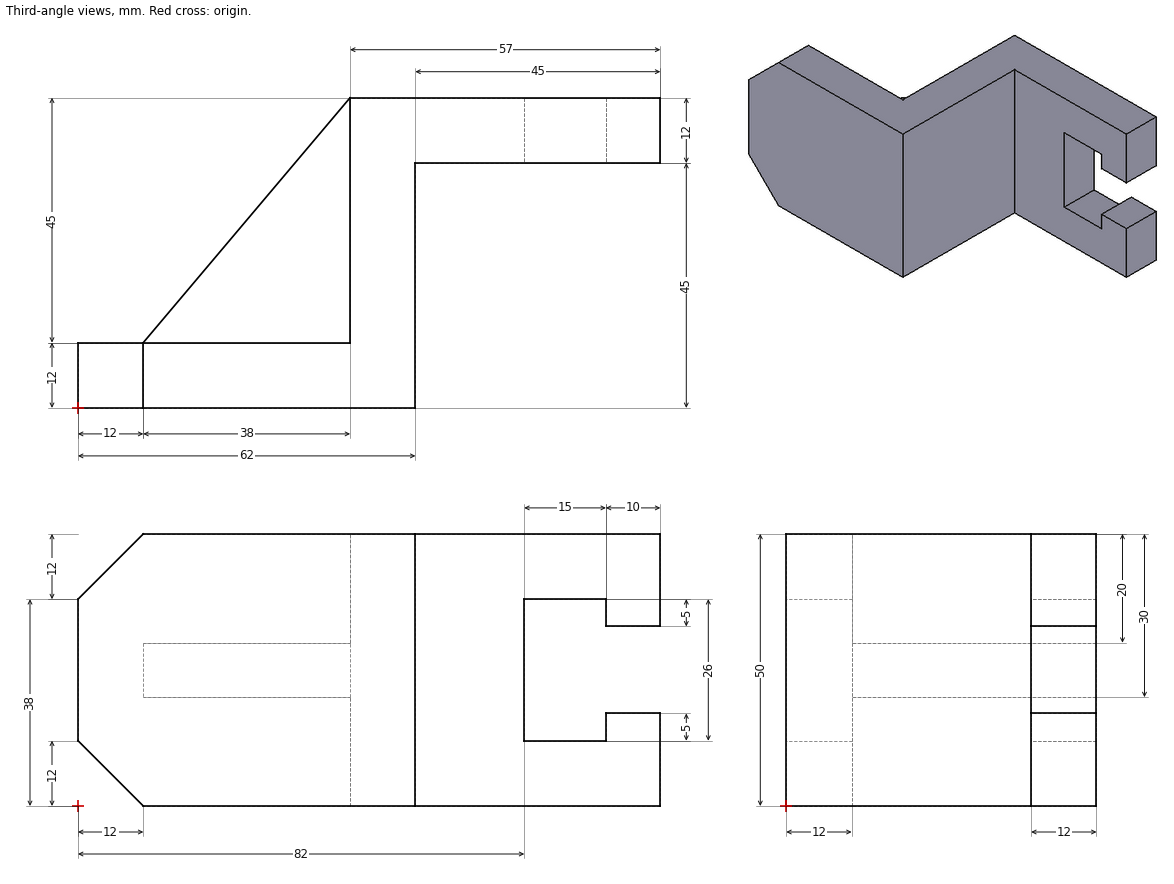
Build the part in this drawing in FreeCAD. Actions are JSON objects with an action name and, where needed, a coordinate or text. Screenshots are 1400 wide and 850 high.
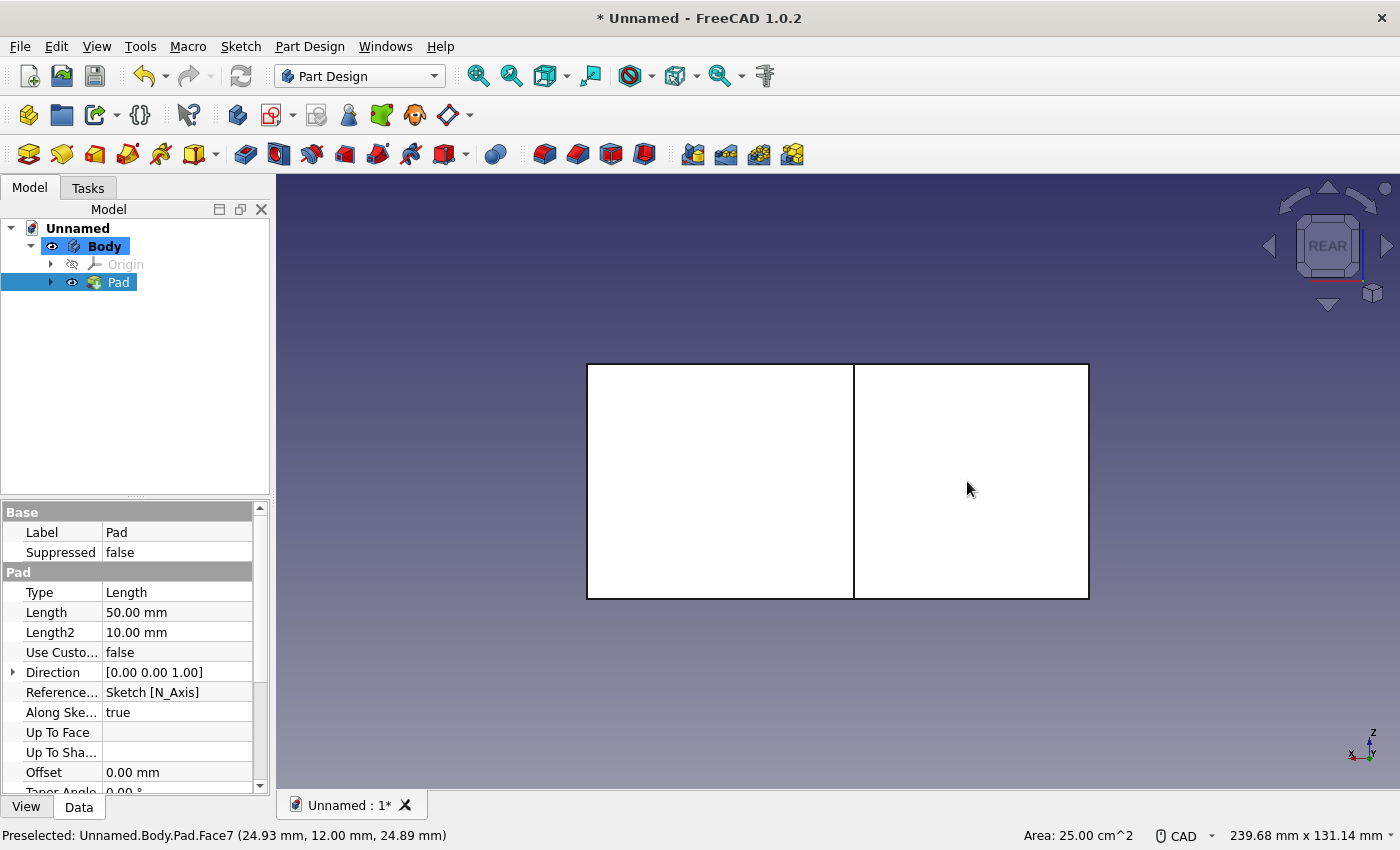
{"action": "left_click", "coordinate": [270, 116]}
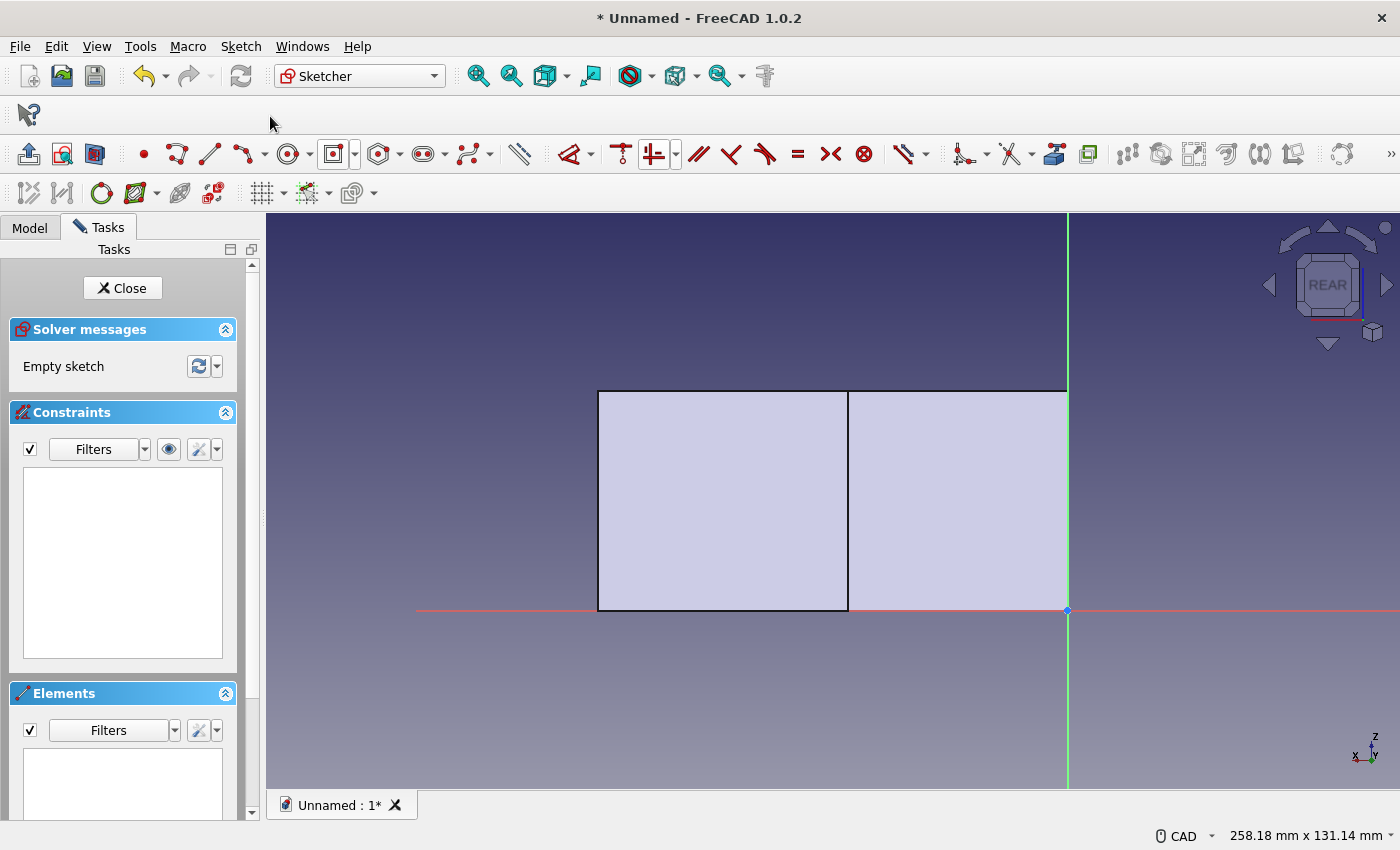
{"action": "scroll", "coordinate": [1235, 501], "scroll_direction": "up", "scroll_amount": 3}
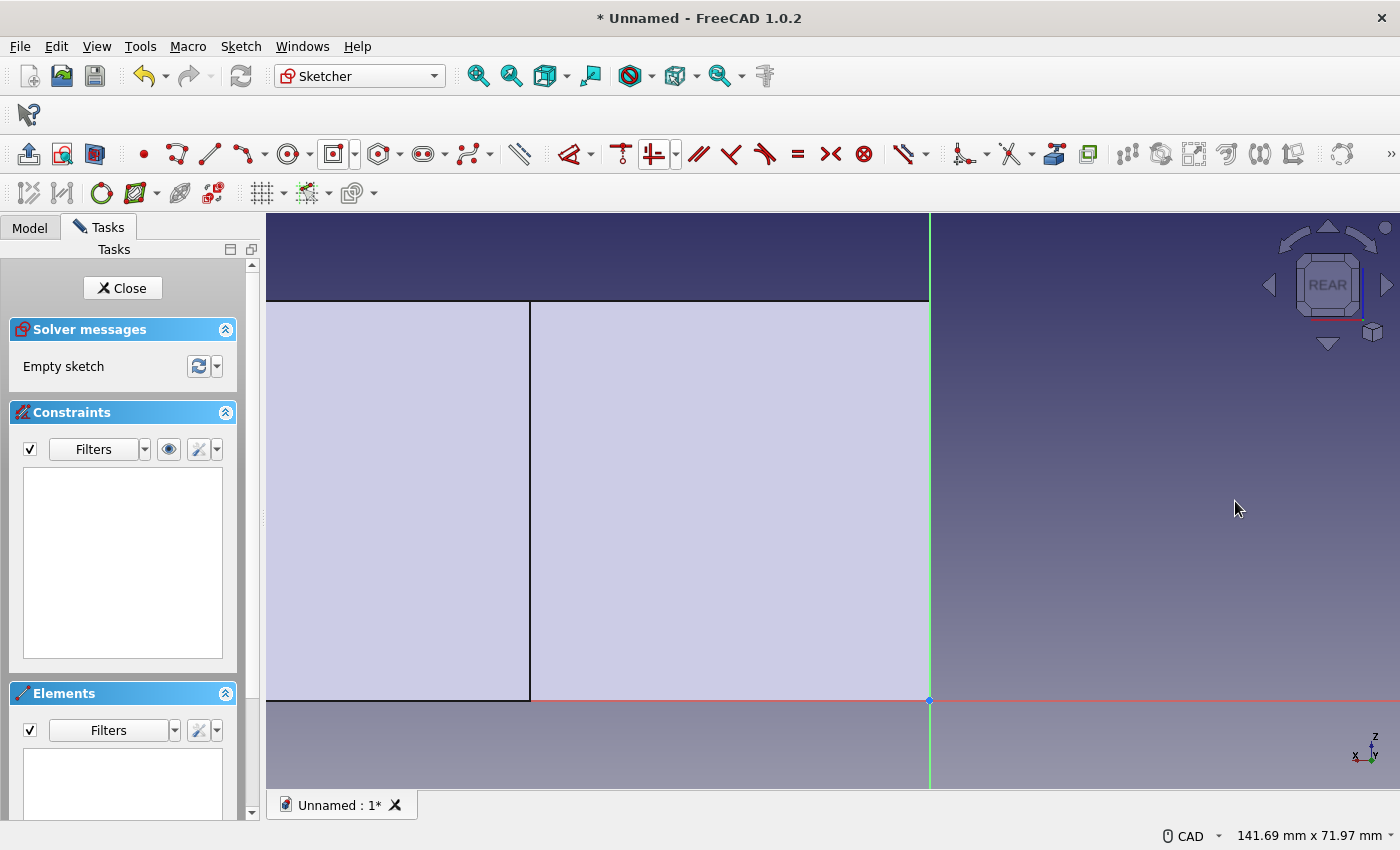
{"action": "left_click", "coordinate": [177, 154]}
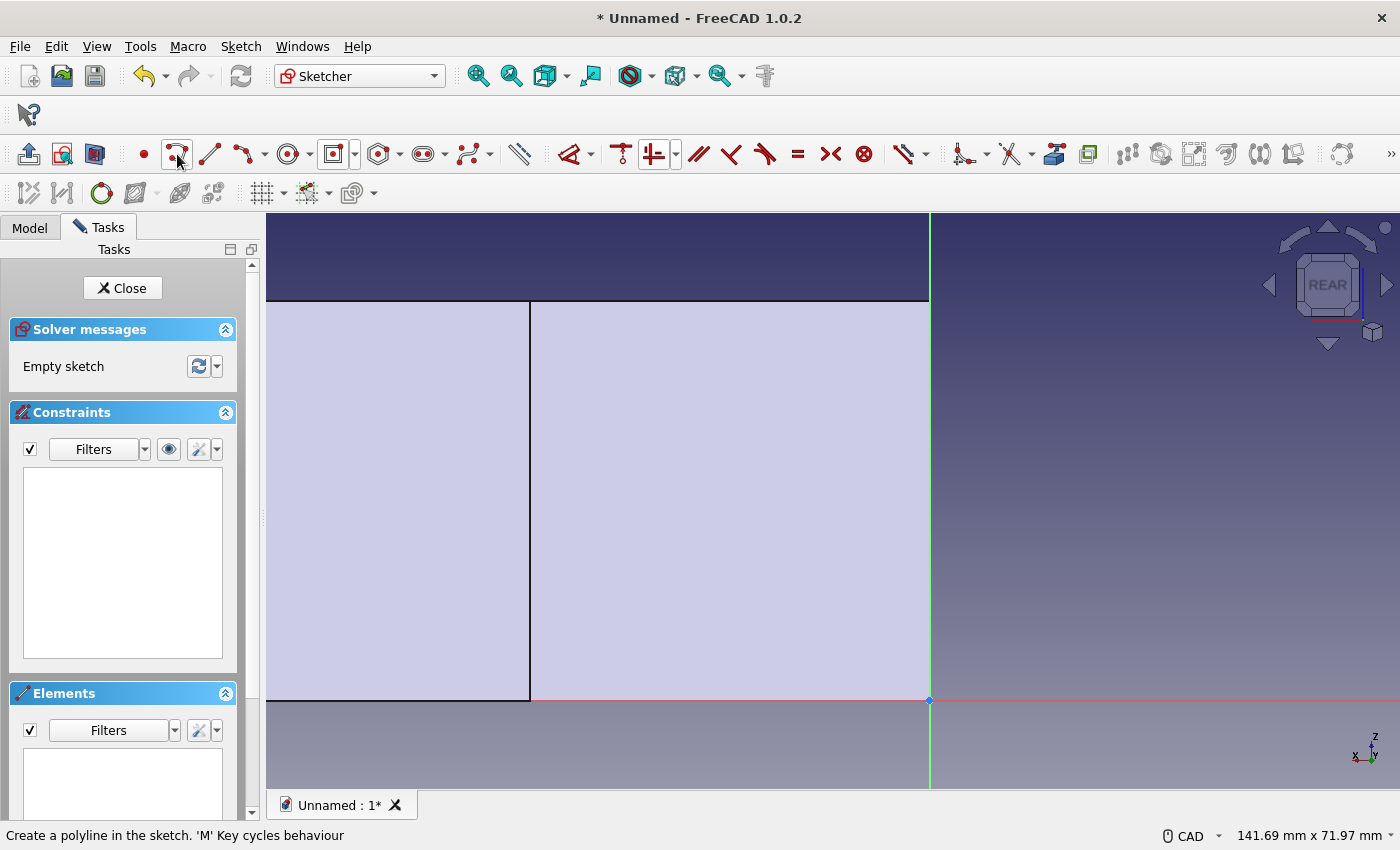
{"action": "left_click", "coordinate": [930, 701]}
{"action": "left_click", "coordinate": [921, 605]}
{"action": "left_click", "coordinate": [834, 692]}
{"action": "left_click", "coordinate": [930, 701]}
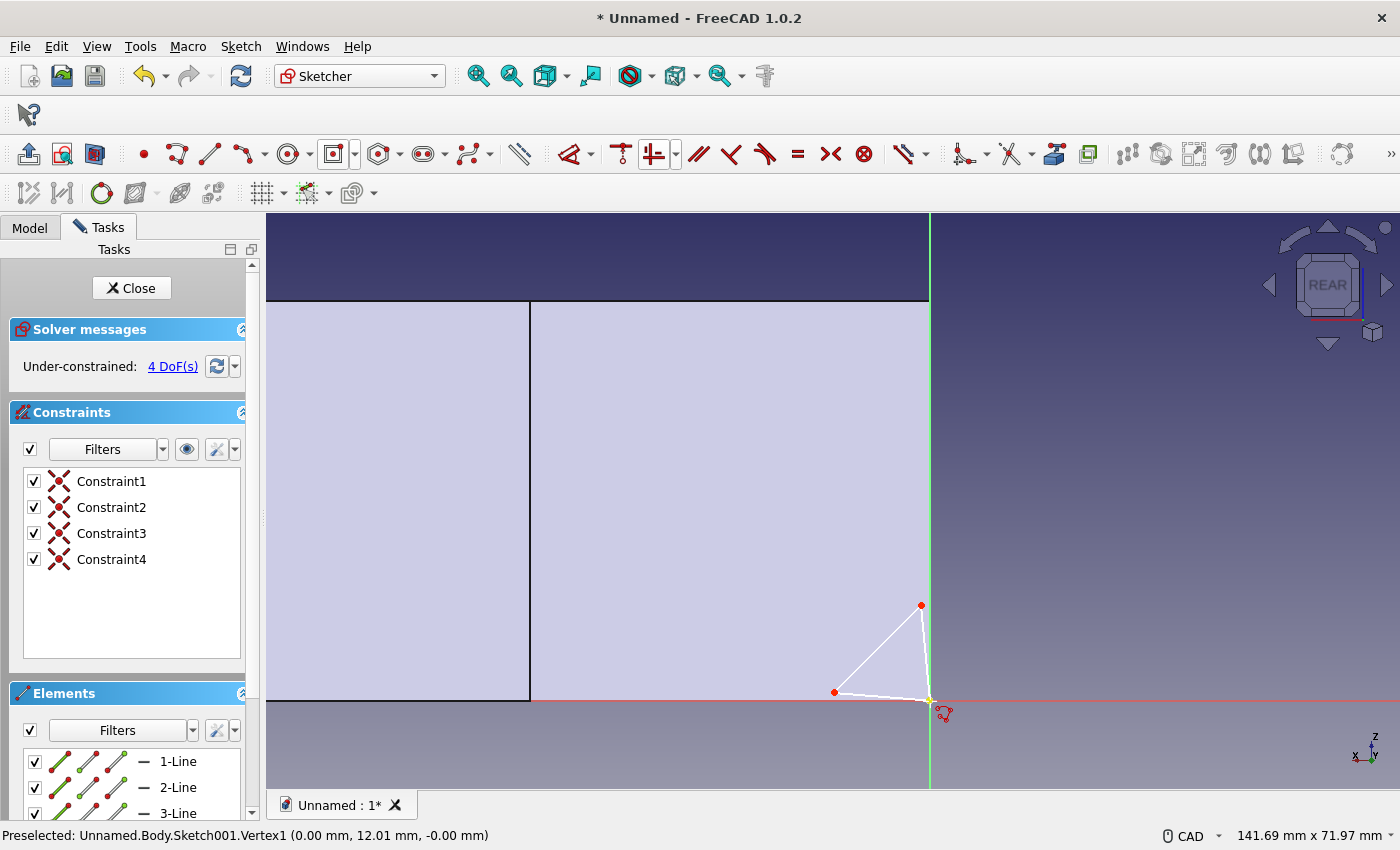
{"action": "left_click", "coordinate": [930, 397]}
{"action": "left_click", "coordinate": [921, 301]}
{"action": "left_click", "coordinate": [834, 301]}
{"action": "left_click", "coordinate": [930, 398]}
{"action": "key", "text": "Escape"}
{"action": "key", "text": "Escape"}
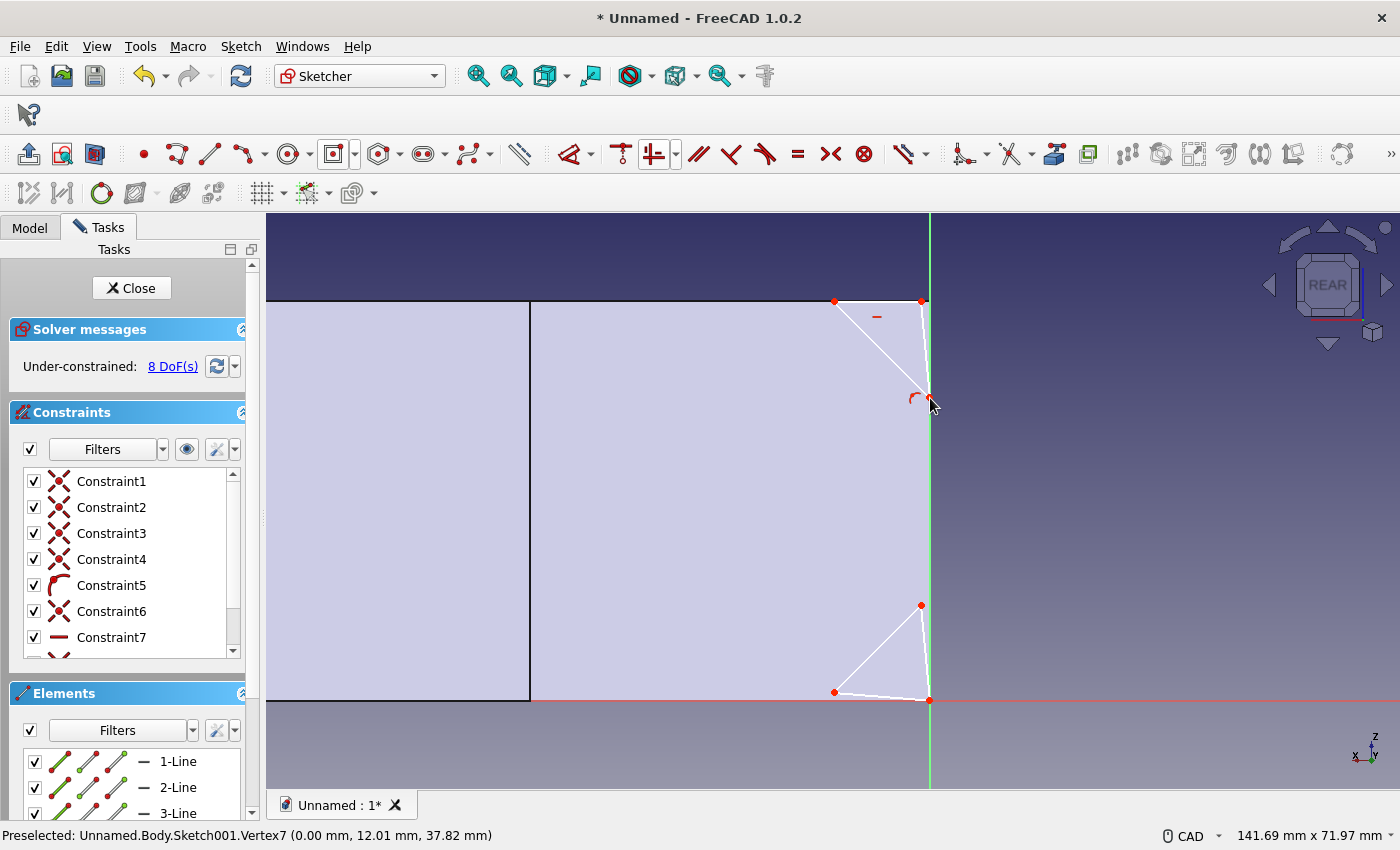
{"action": "left_click", "coordinate": [927, 672]}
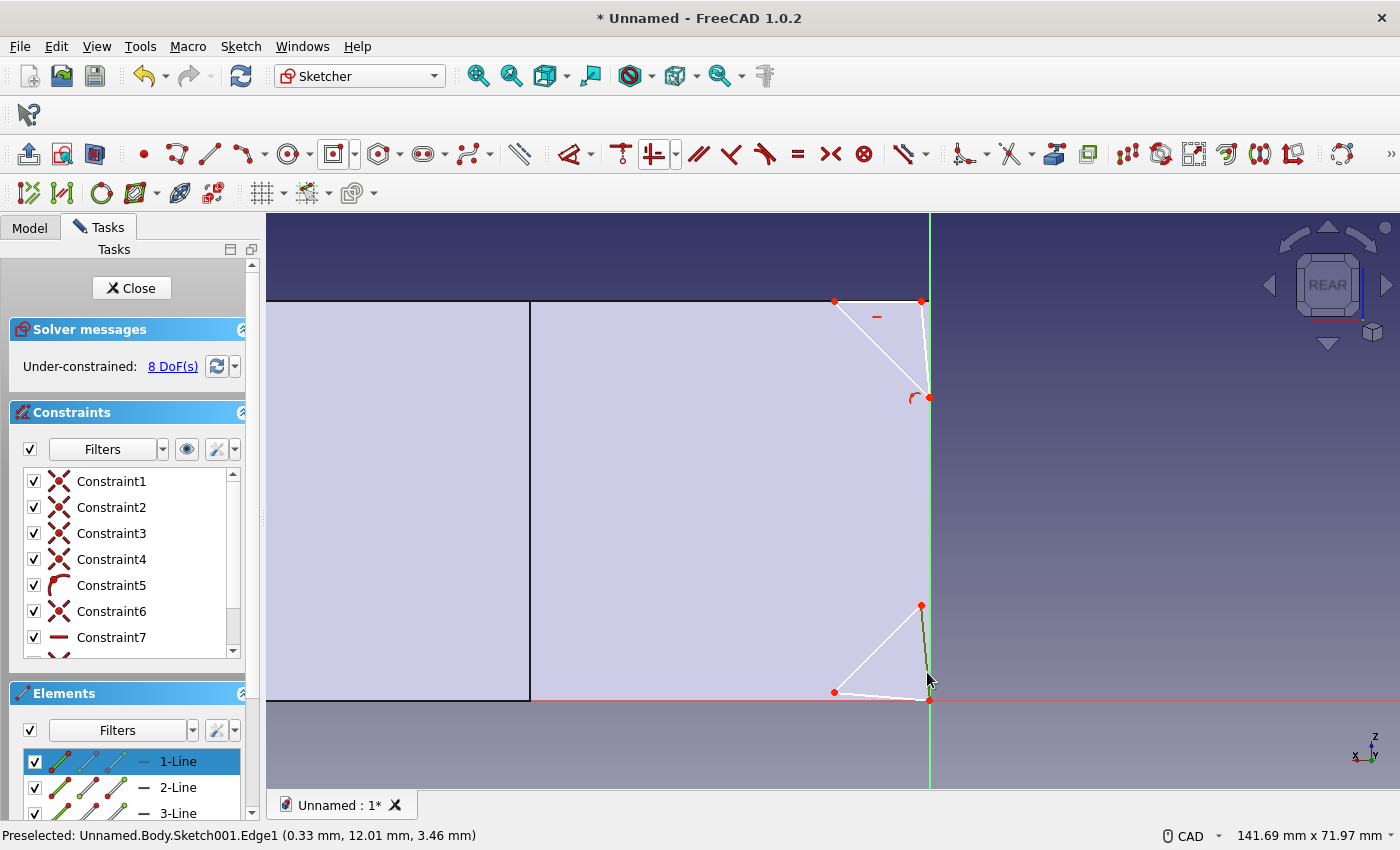
{"action": "left_click", "coordinate": [676, 154]}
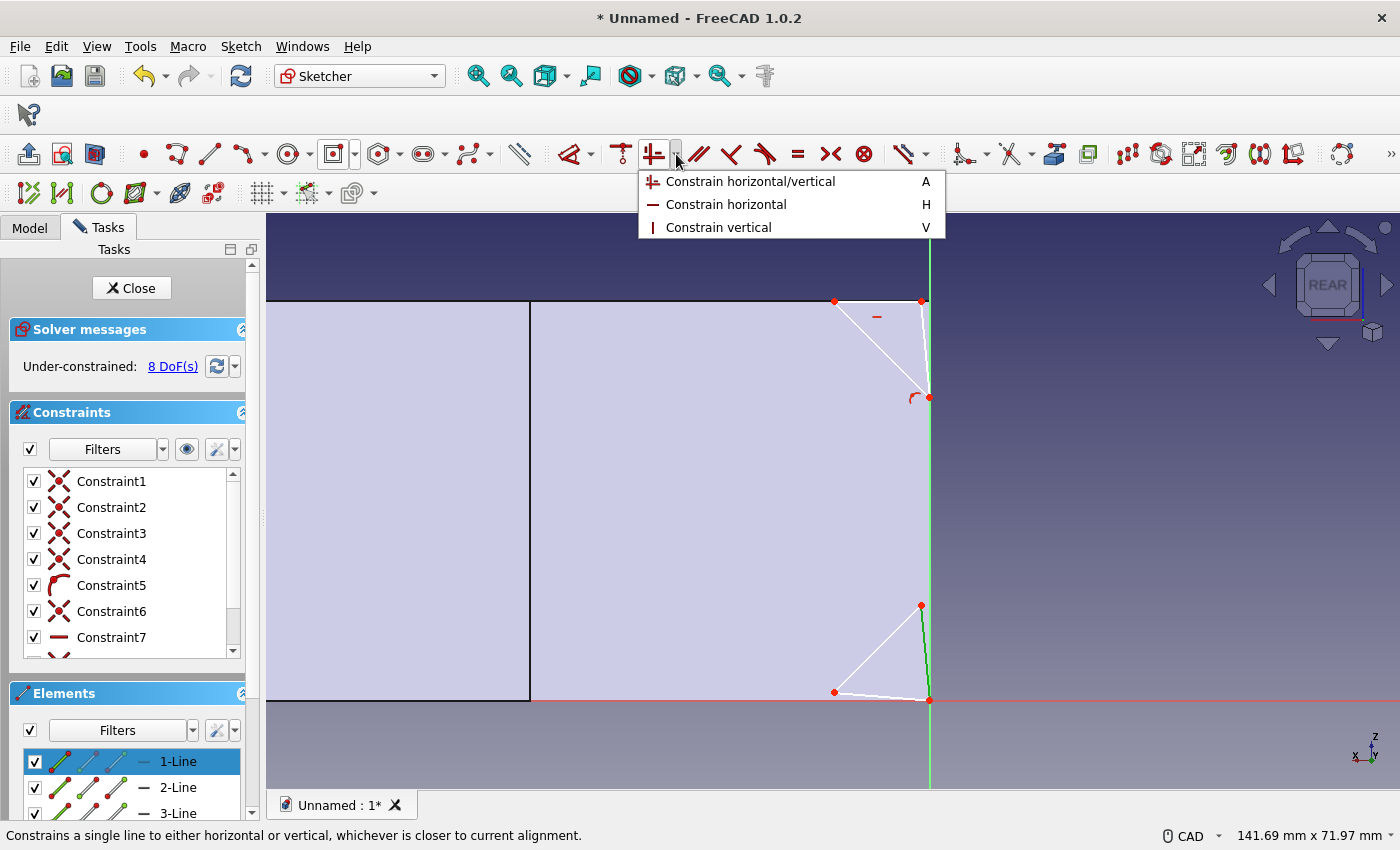
{"action": "left_click", "coordinate": [792, 228]}